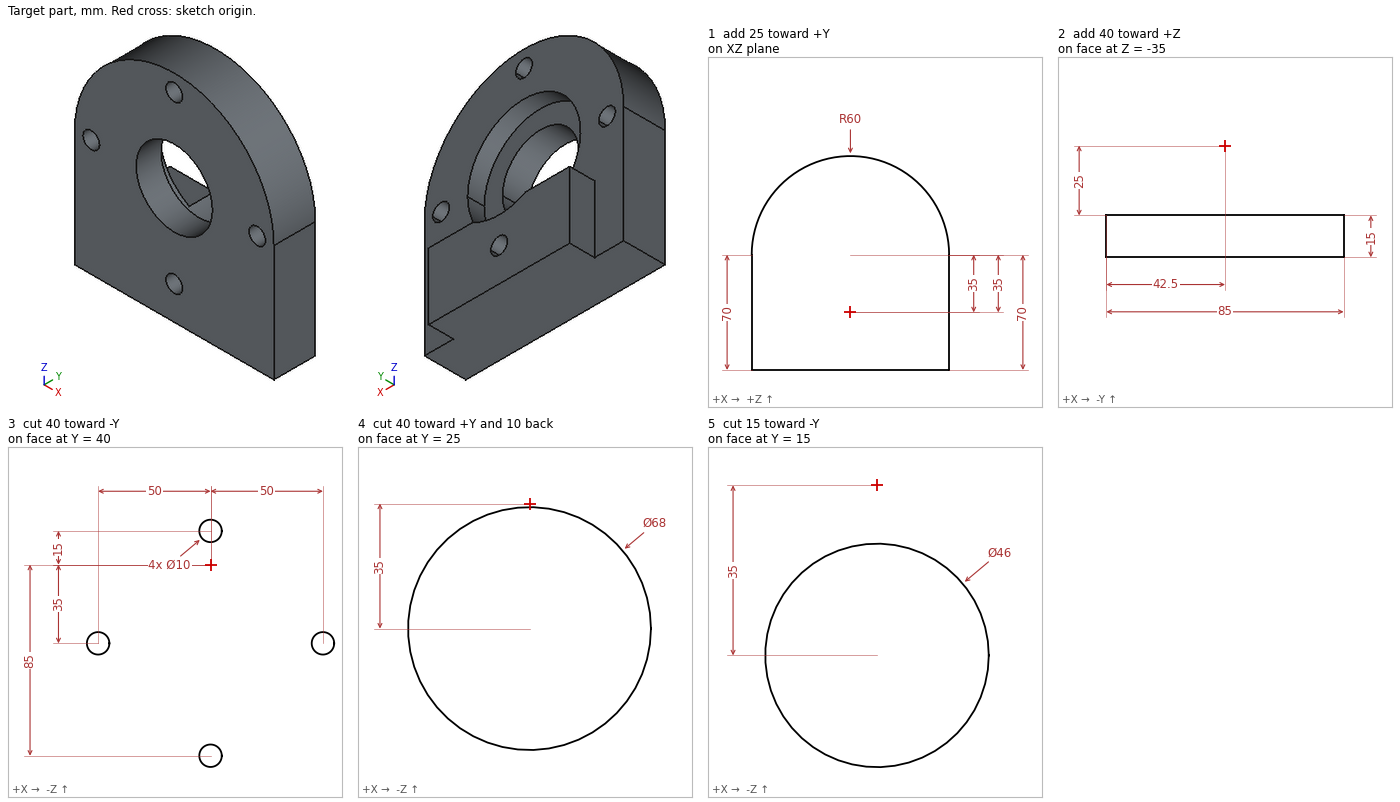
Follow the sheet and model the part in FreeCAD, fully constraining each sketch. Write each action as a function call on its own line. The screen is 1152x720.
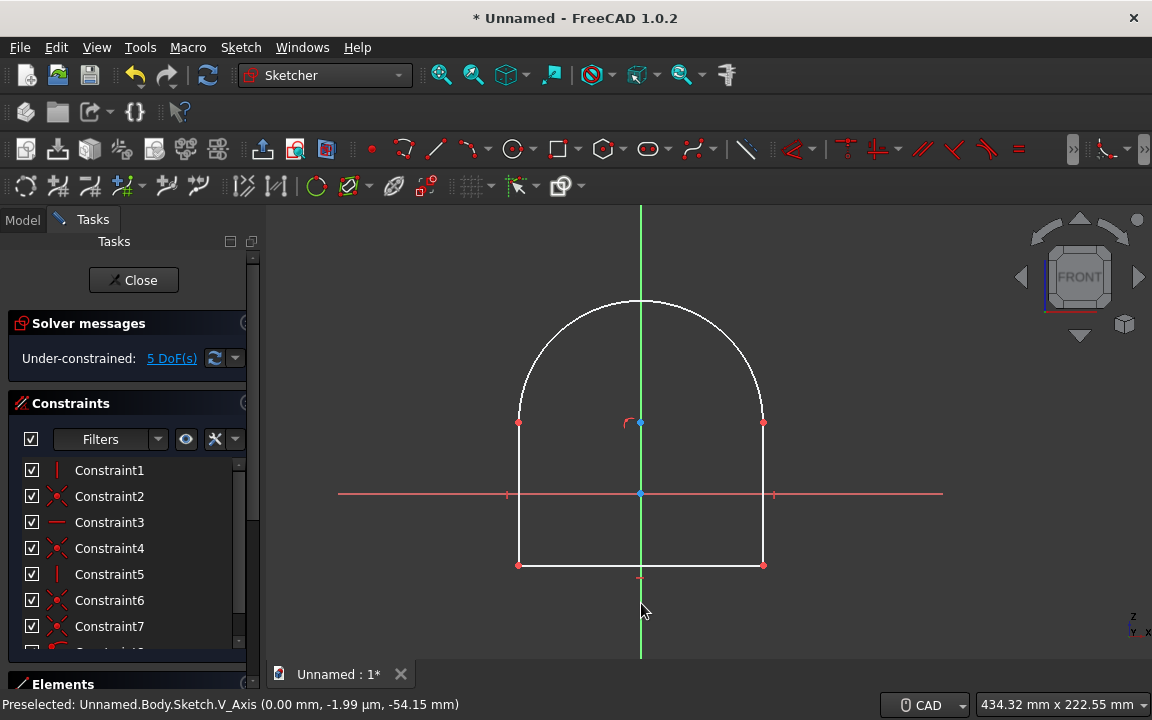
key(d)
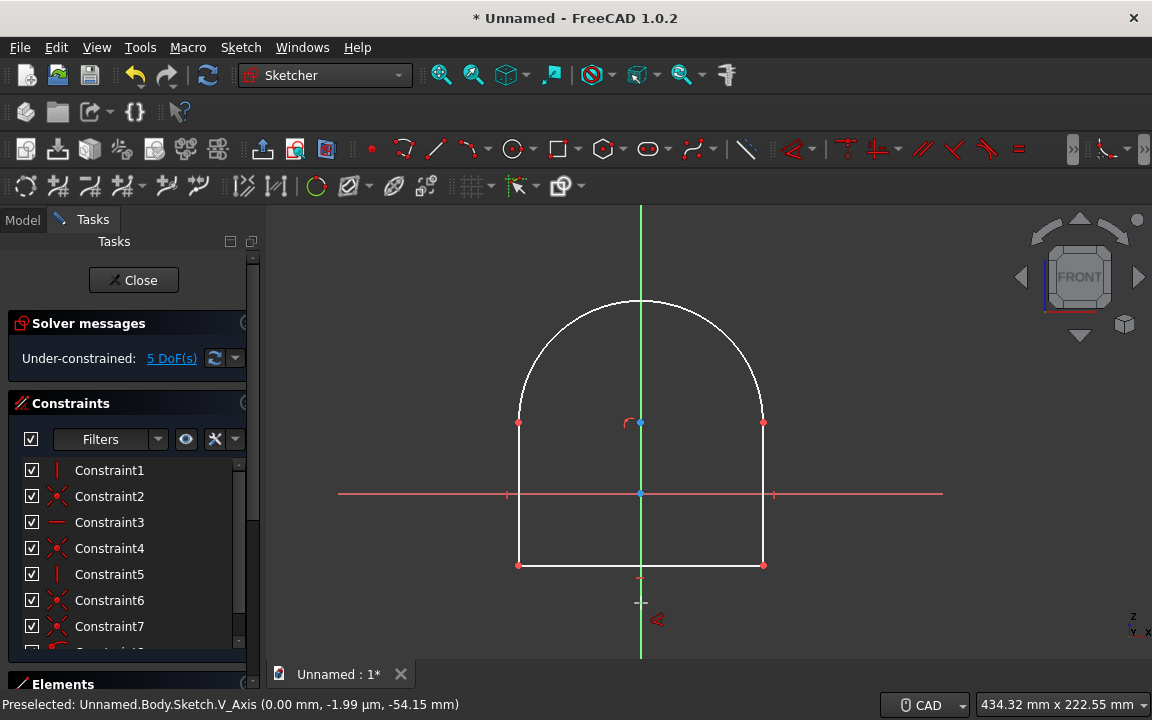
click(713, 324)
click(732, 298)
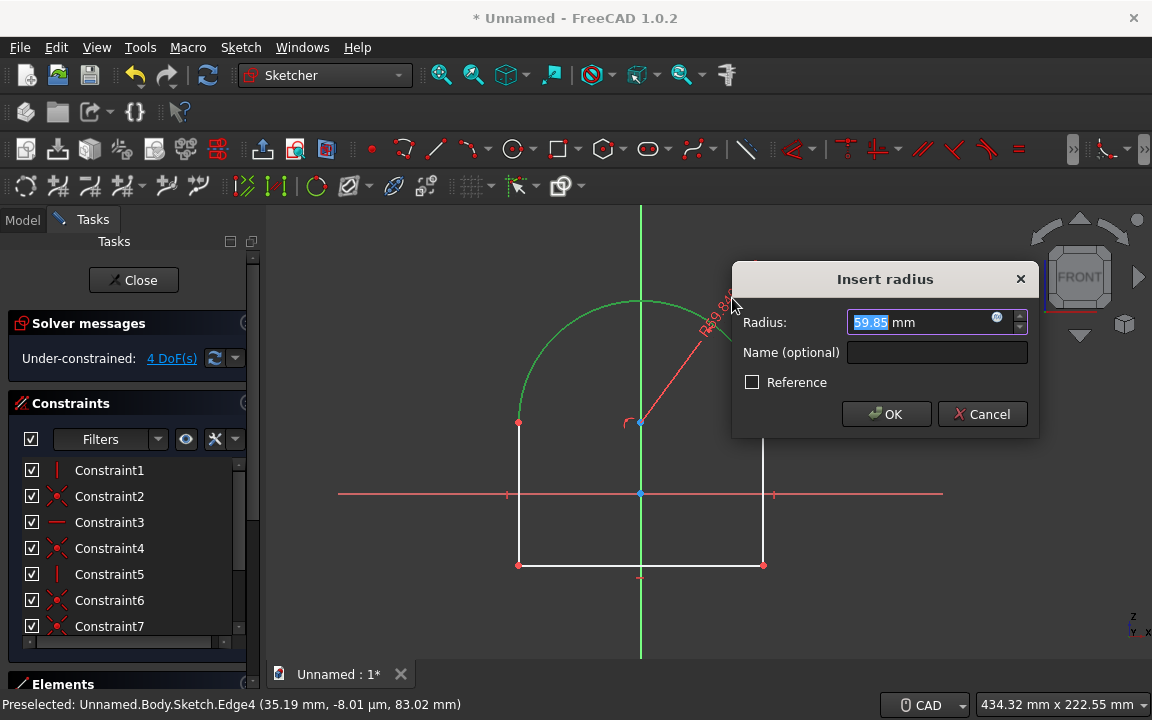
text(60)
key(Return)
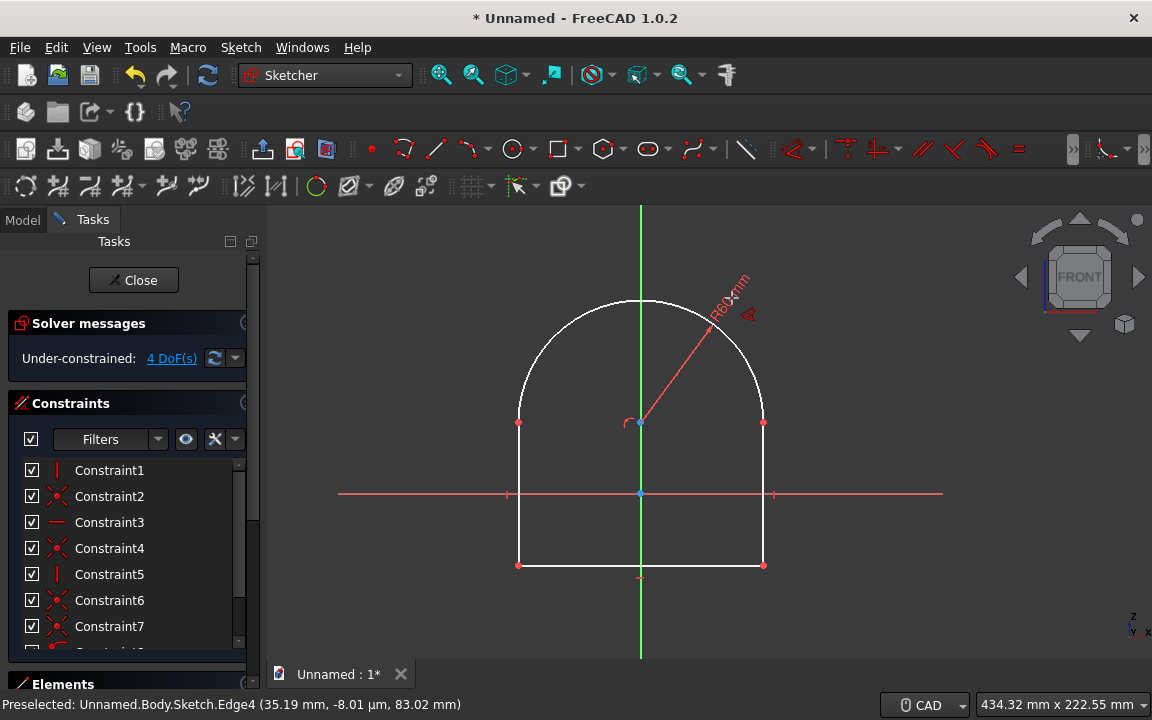
click(763, 466)
click(797, 462)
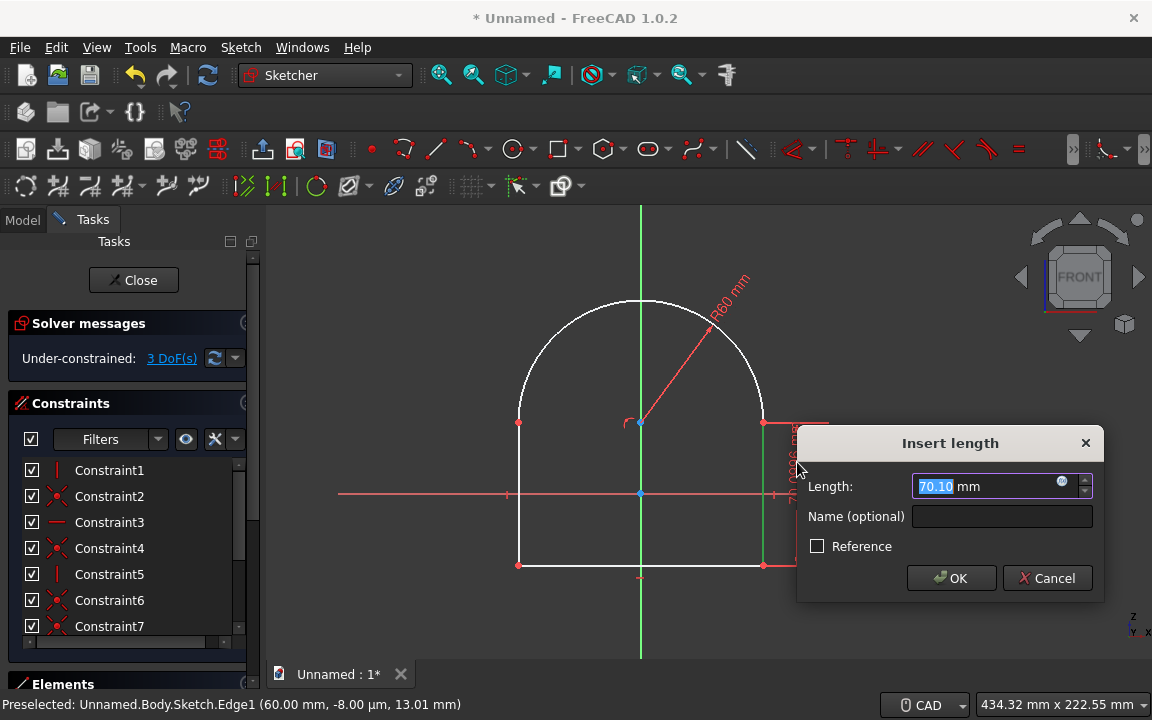
text(70)
key(Return)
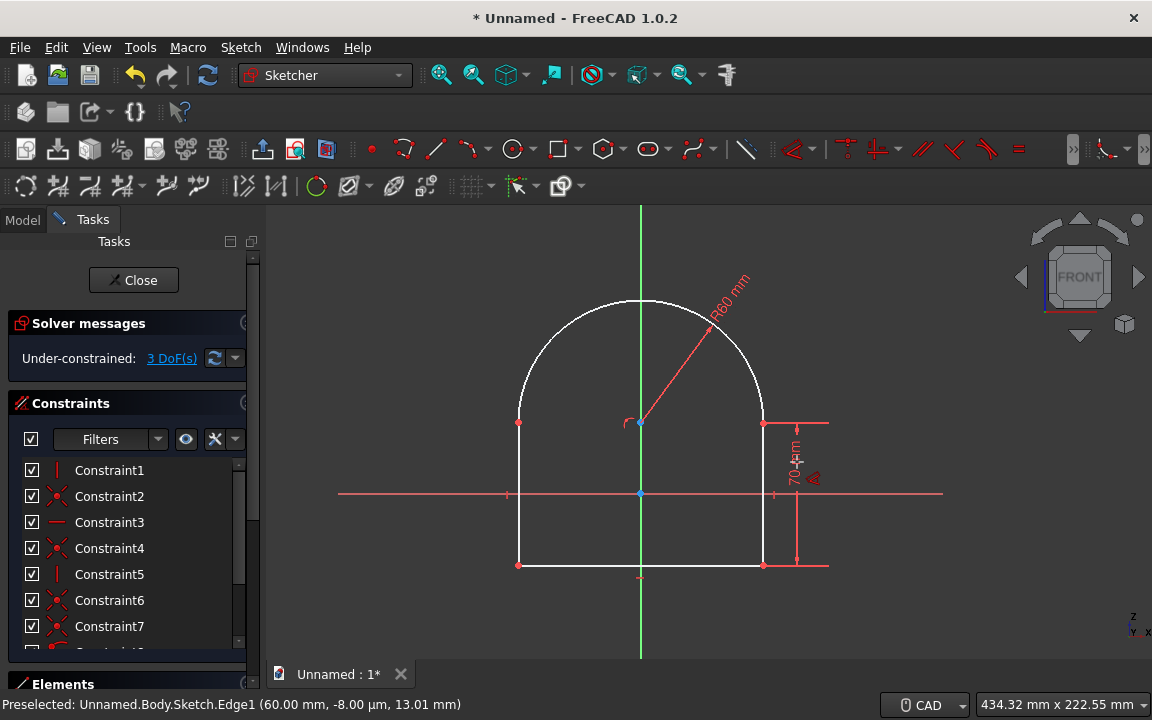
click(519, 523)
click(485, 462)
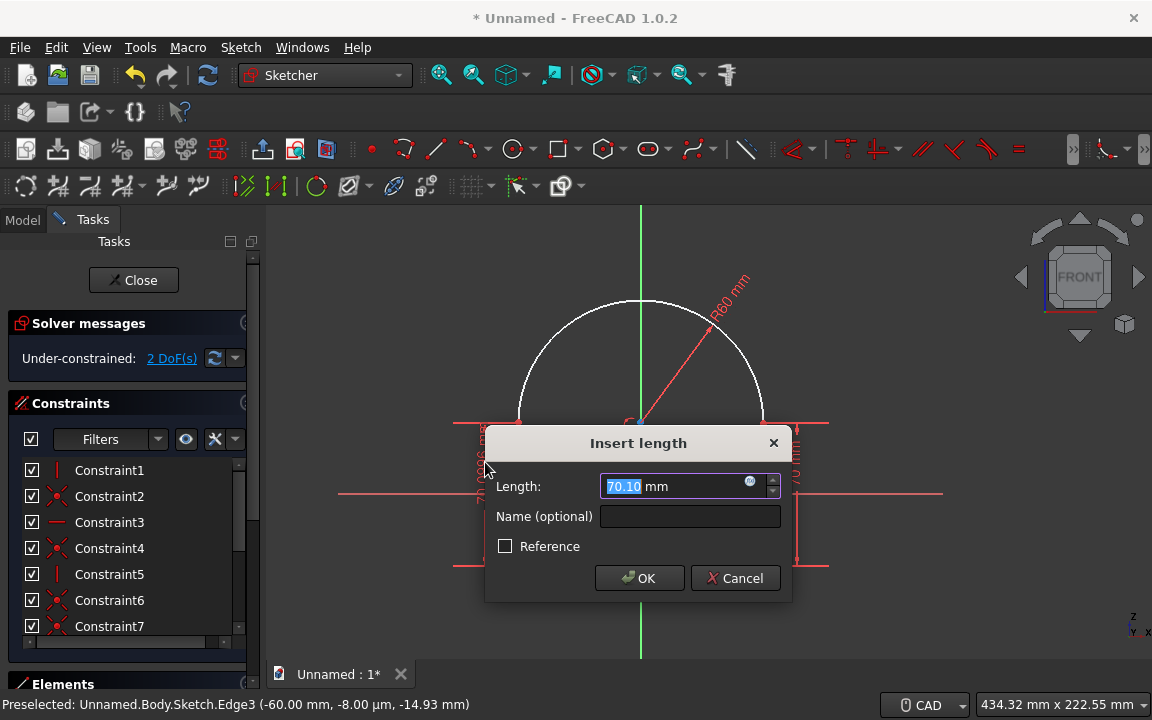
text(70)
key(Return)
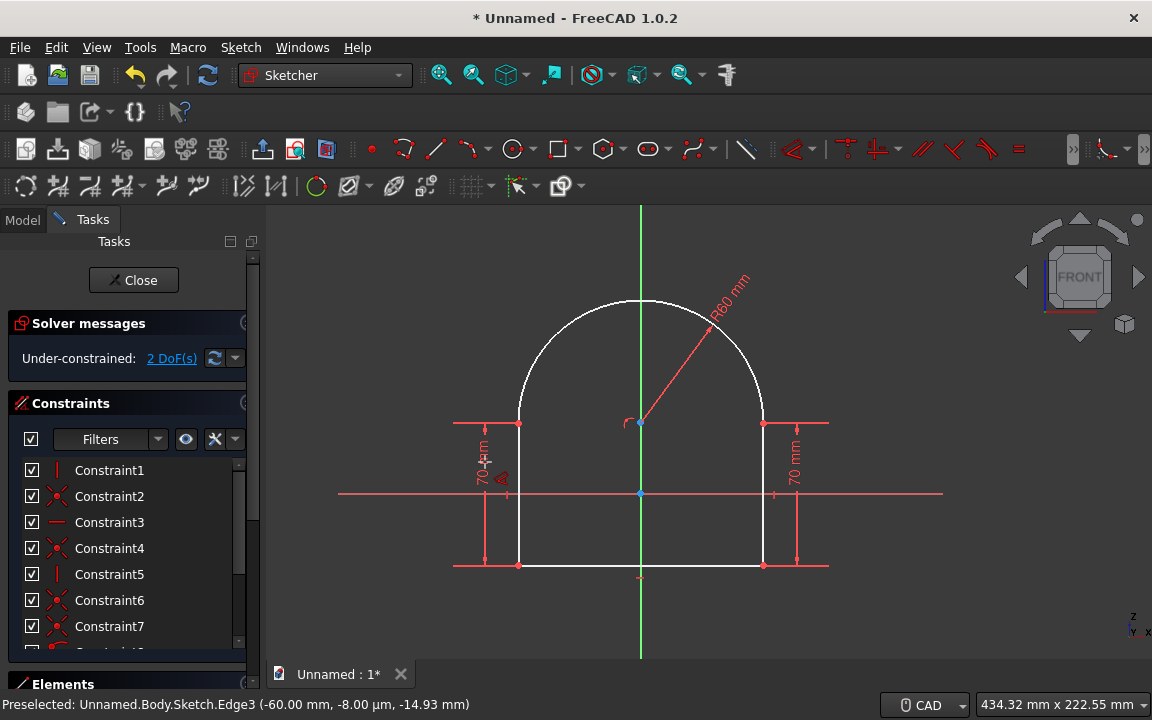
click(763, 423)
click(797, 434)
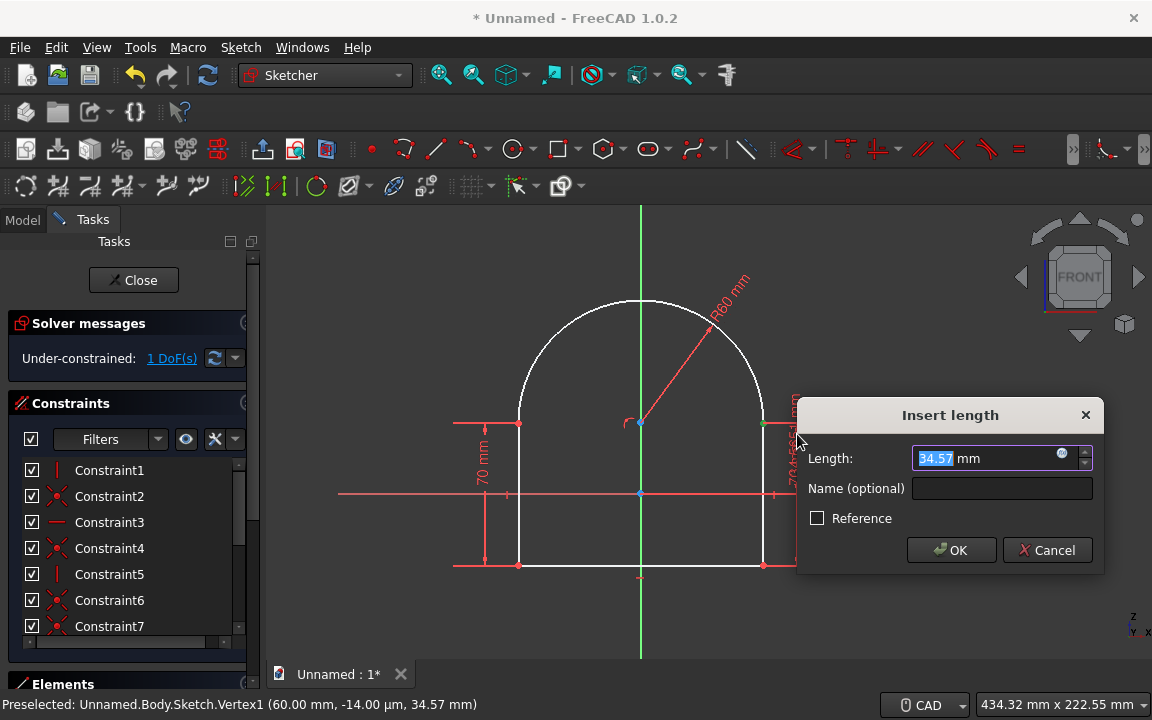
text(35)
key(Return)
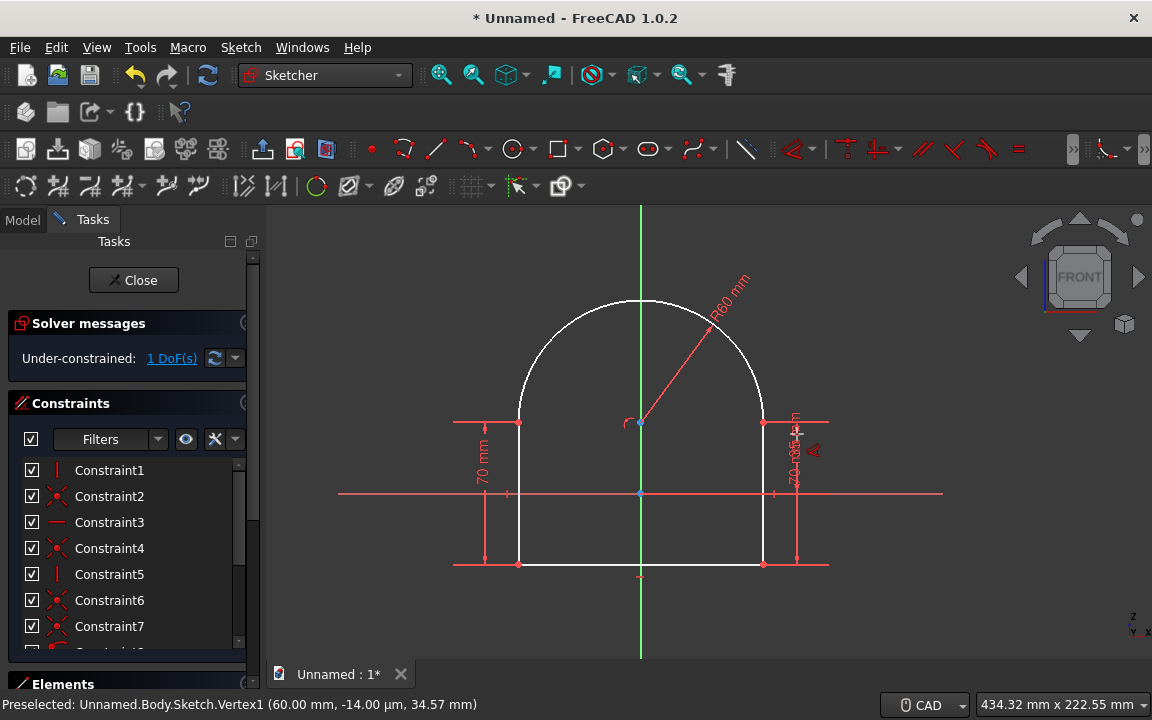
click(641, 423)
click(675, 458)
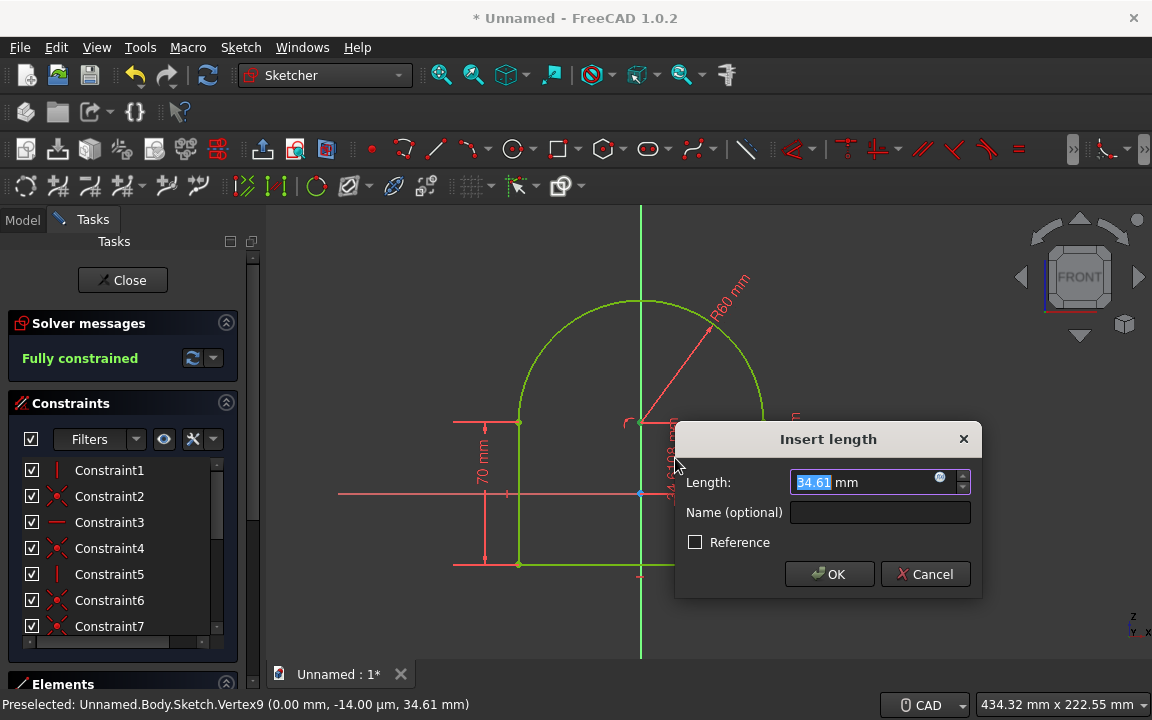
text(35)
key(Return)
key(Escape)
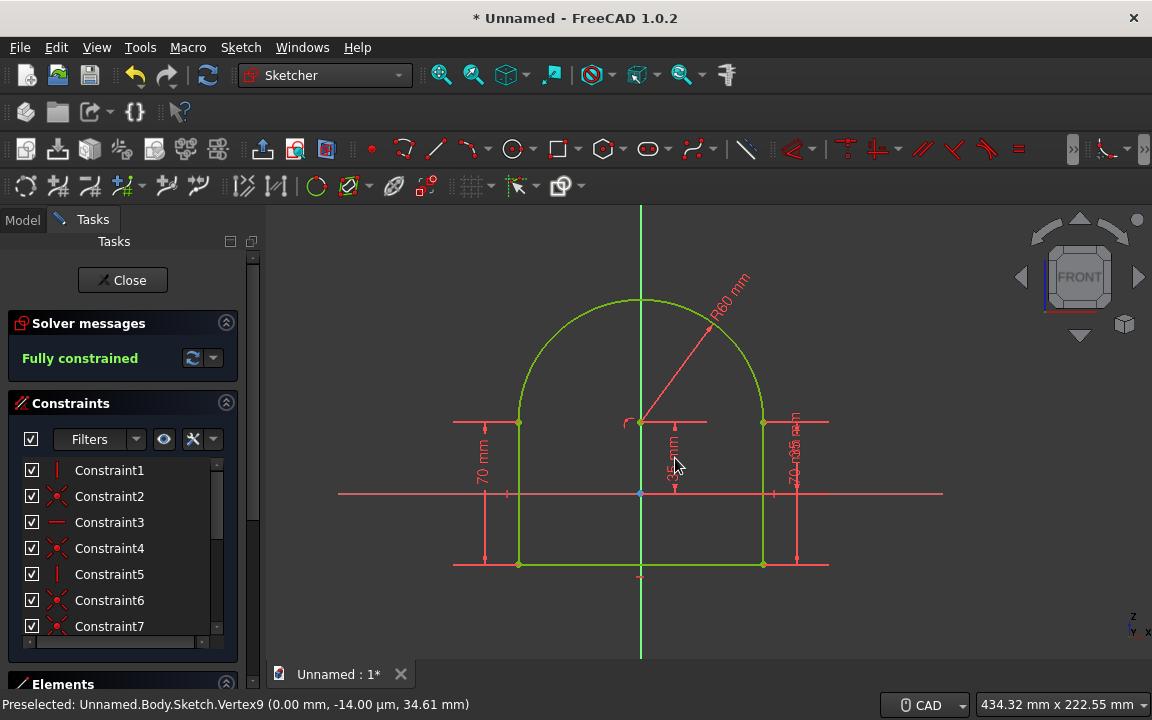
click(123, 280)